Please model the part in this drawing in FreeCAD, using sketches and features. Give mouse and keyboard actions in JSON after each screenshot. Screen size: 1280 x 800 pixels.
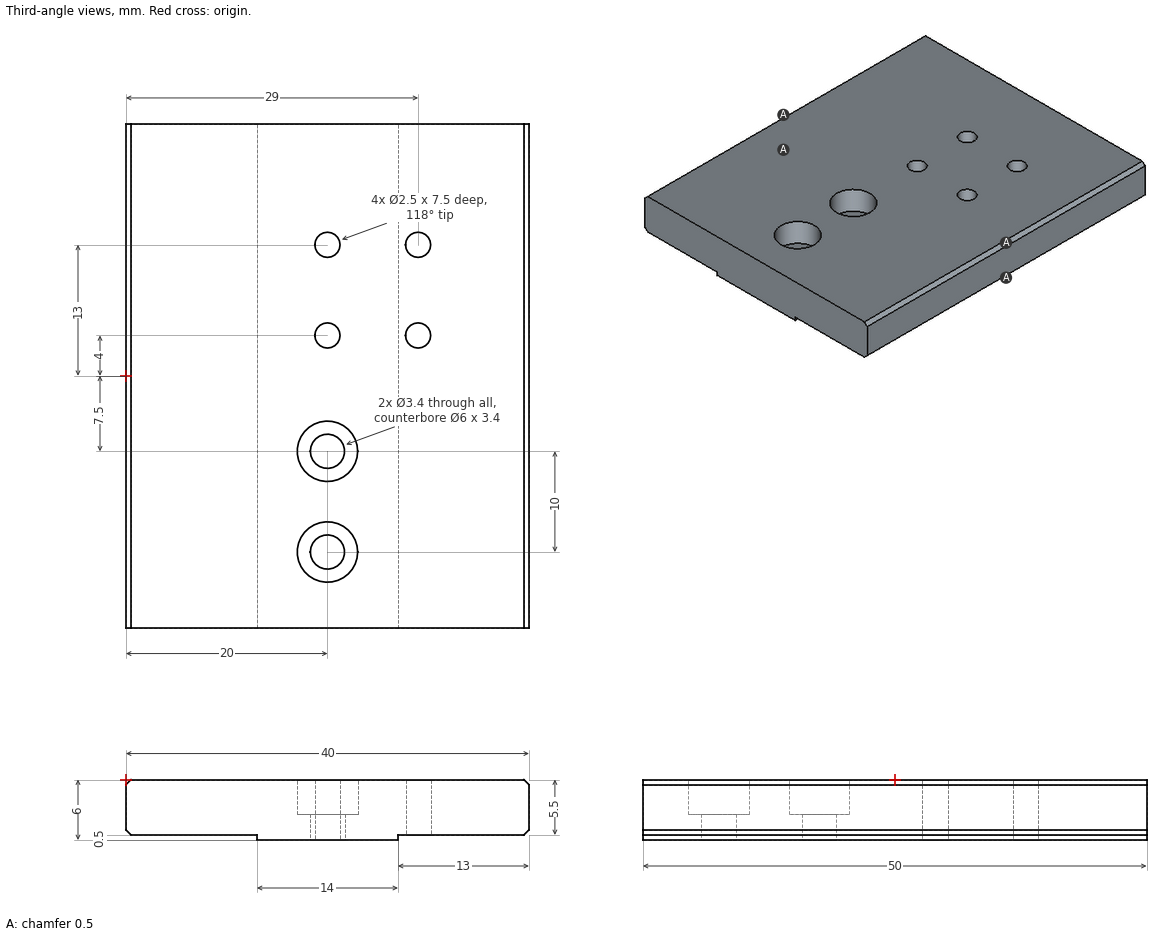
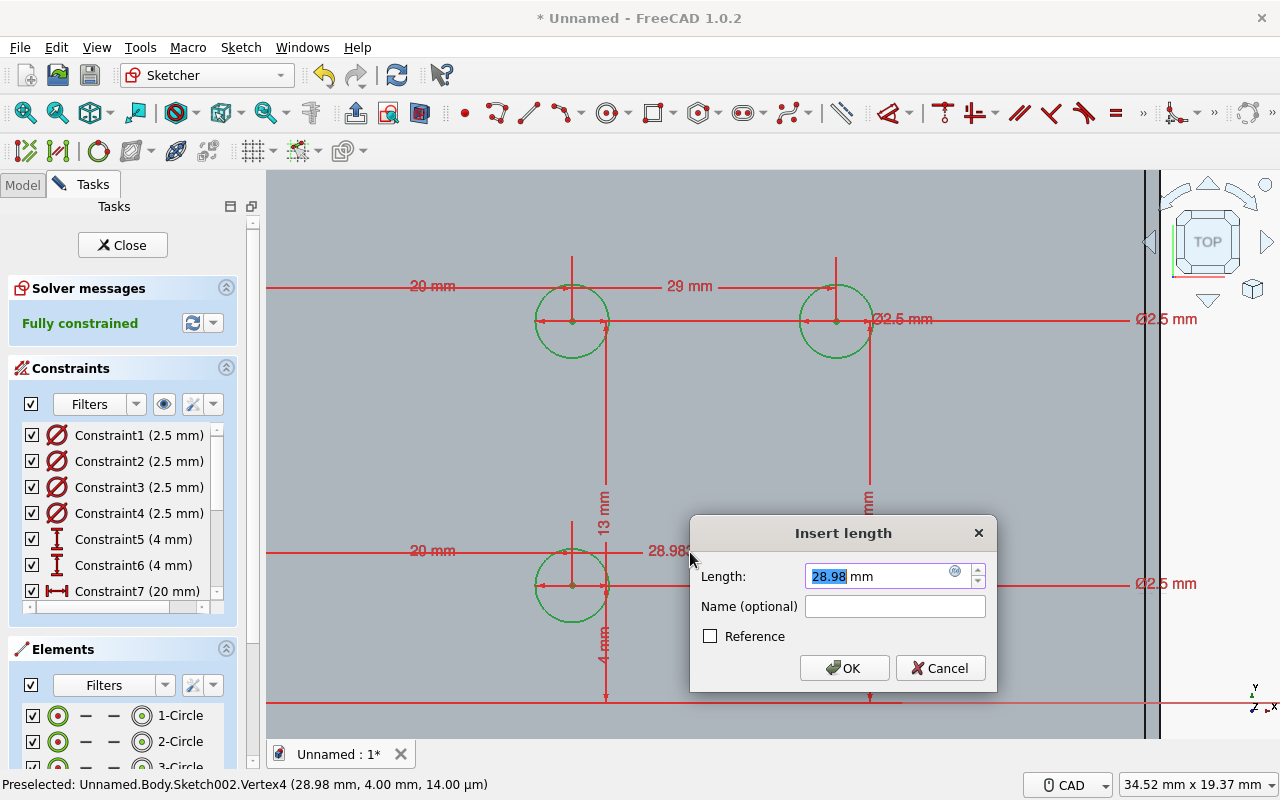
{"action": "type", "text": "29"}
{"action": "key", "text": "Return"}
{"action": "key", "text": "Escape"}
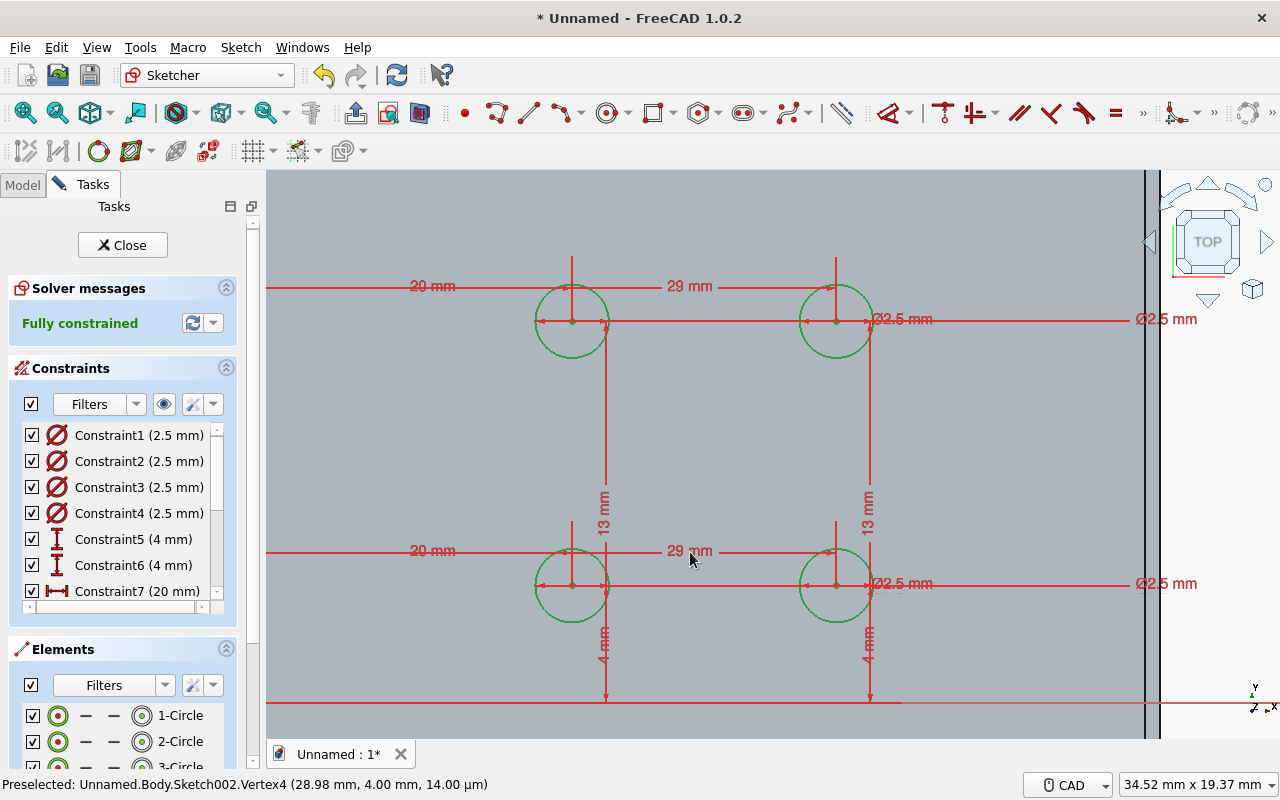
{"action": "left_click", "coordinate": [123, 245]}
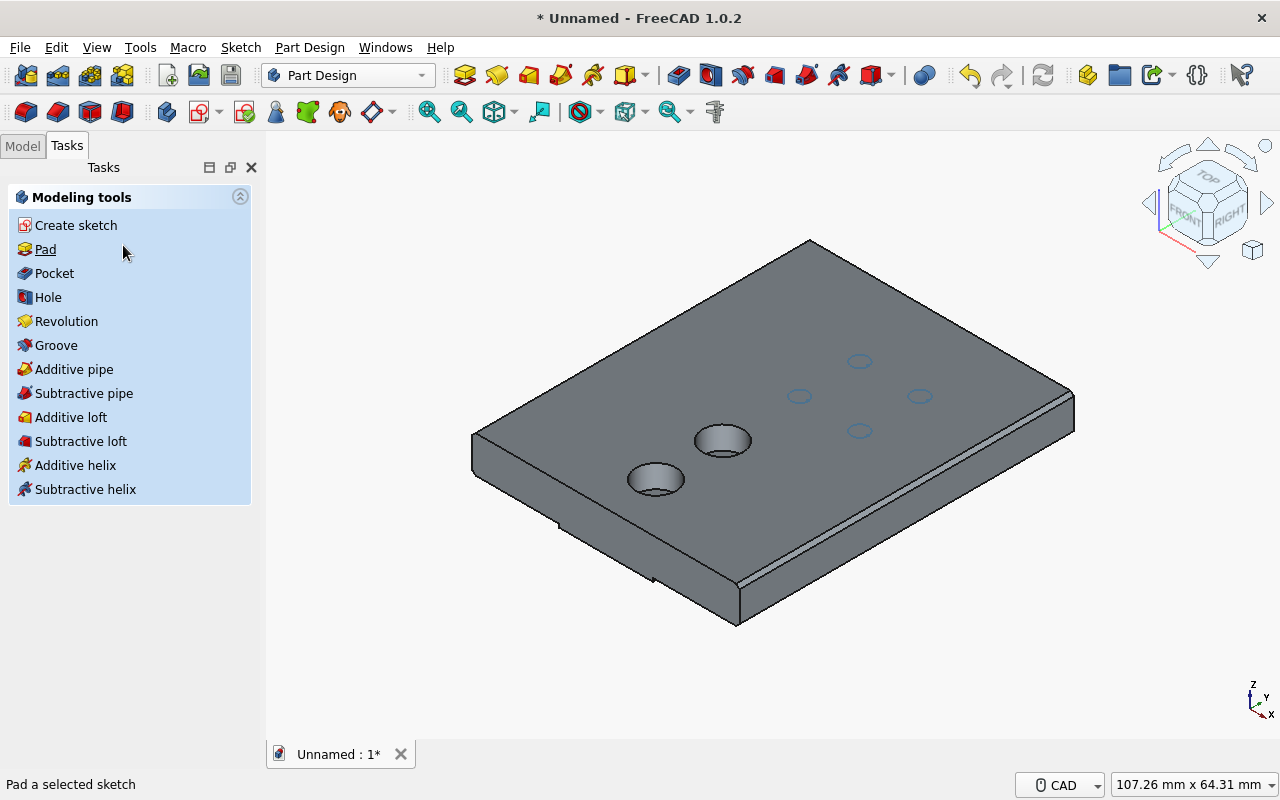
{"action": "left_click", "coordinate": [712, 76]}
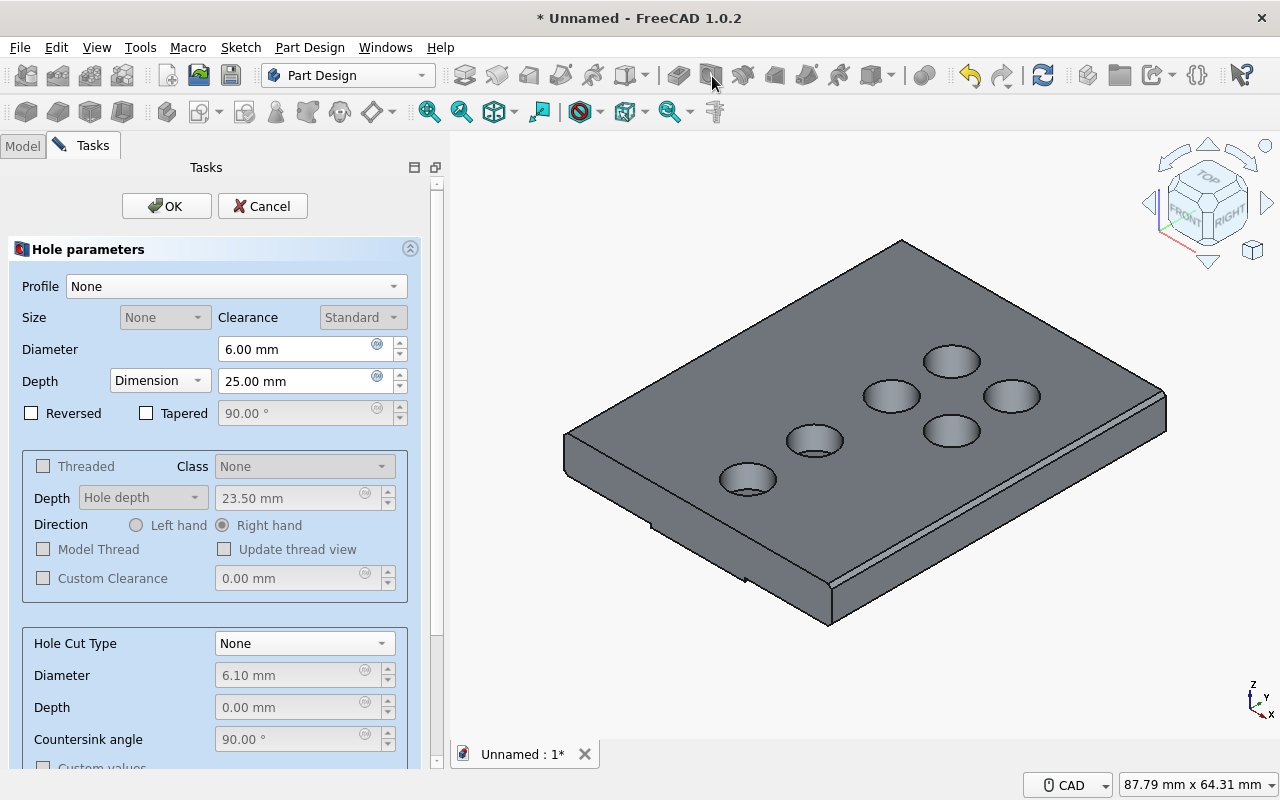
{"action": "triple_click", "coordinate": [305, 349]}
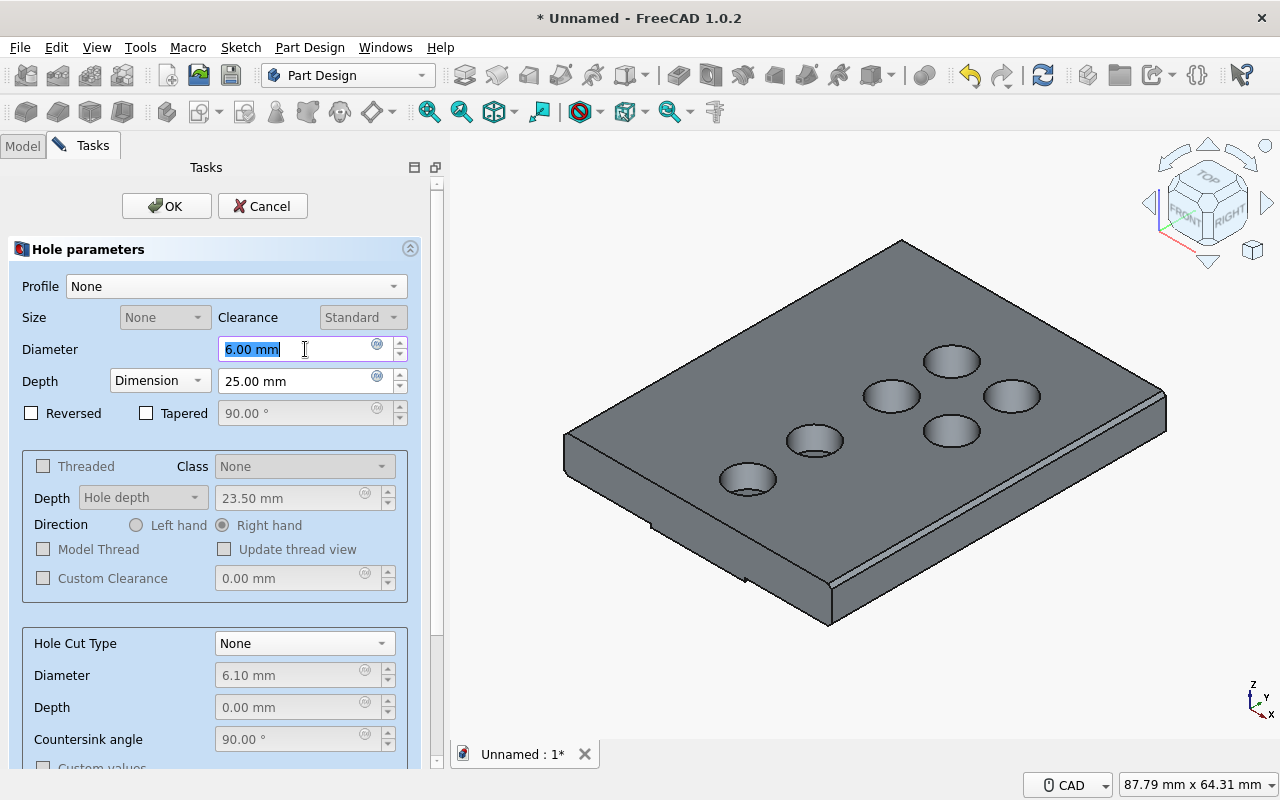
{"action": "type", "text": "2.5"}
{"action": "key", "text": "Tab"}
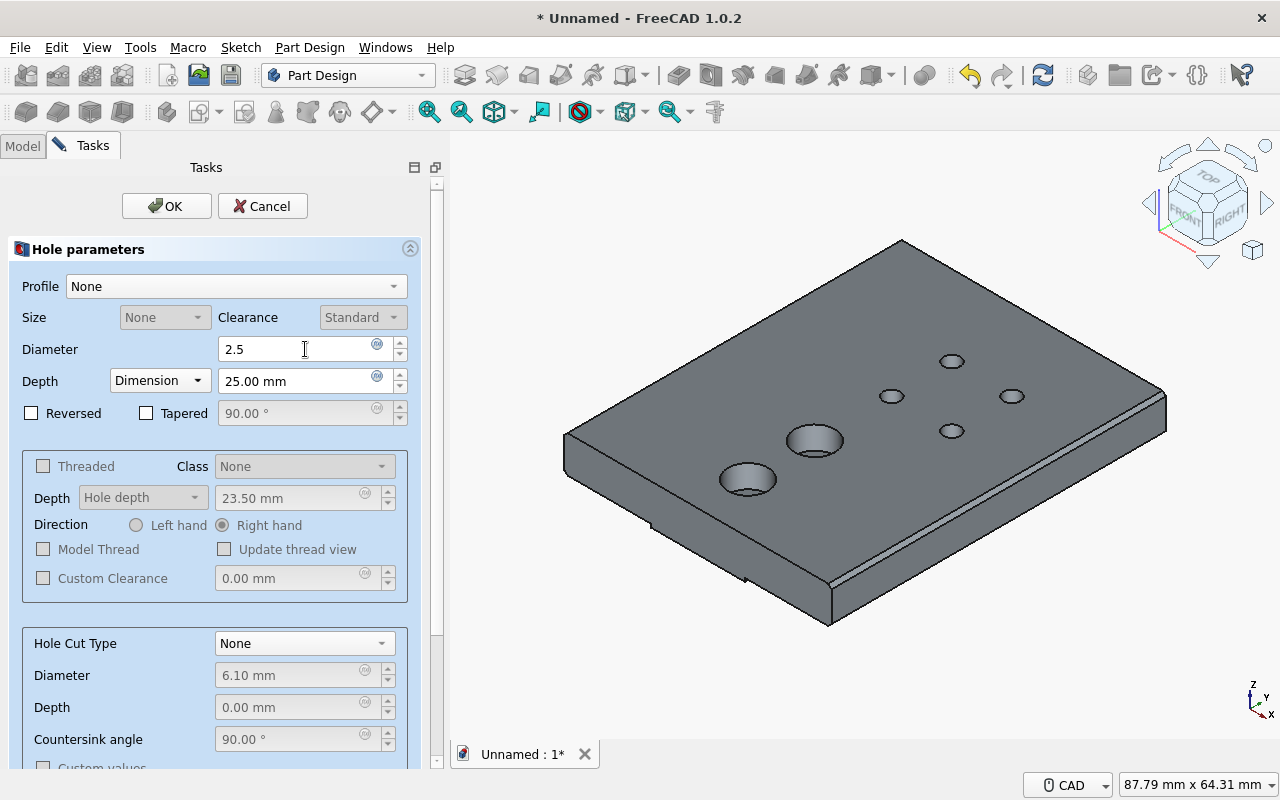
{"action": "triple_click", "coordinate": [305, 381]}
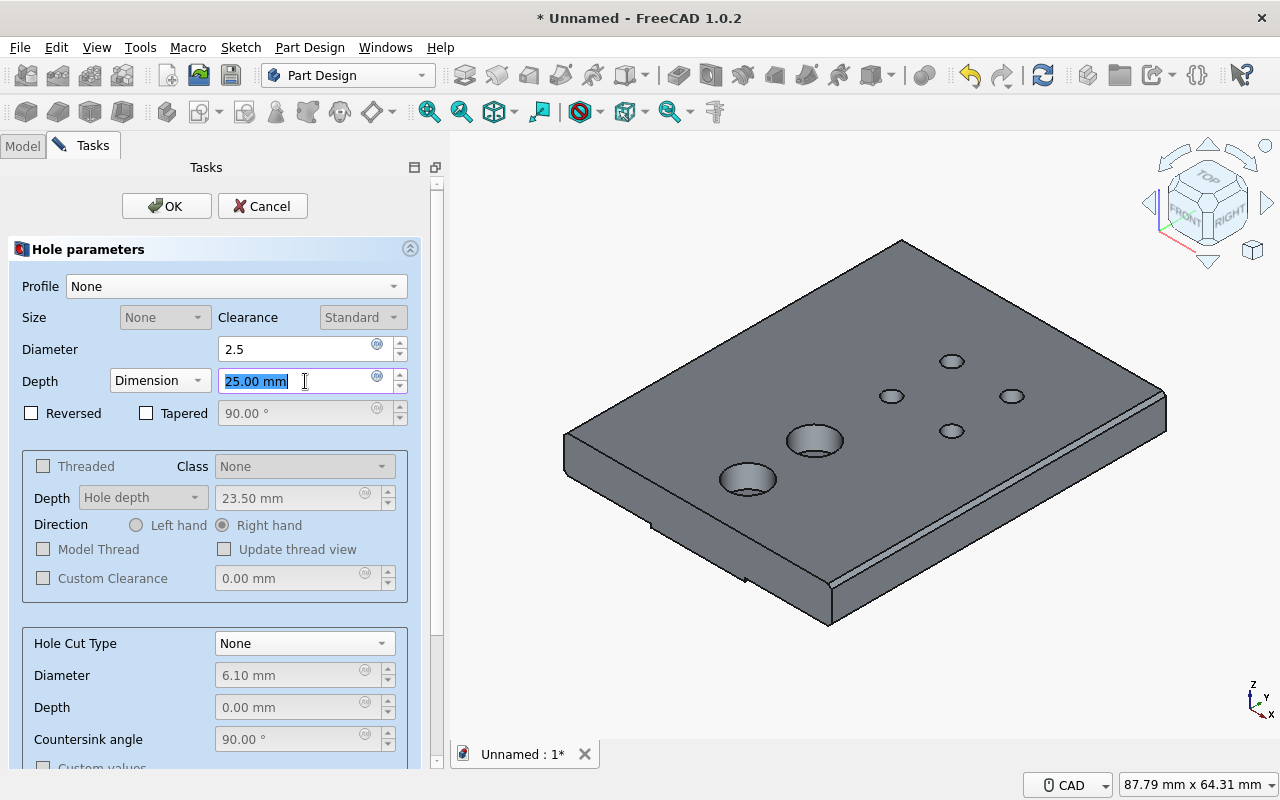
{"action": "type", "text": "7.5"}
{"action": "key", "text": "Tab"}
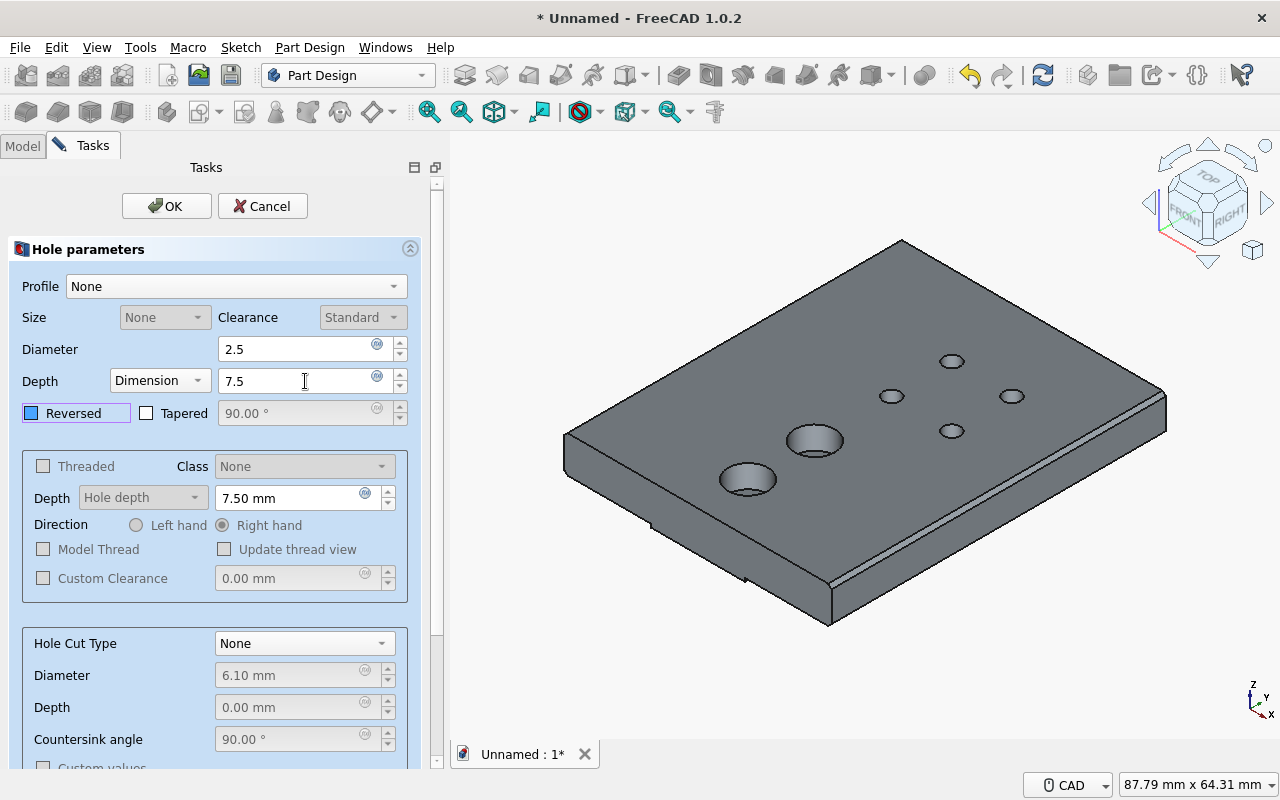
{"action": "left_click", "coordinate": [167, 206]}